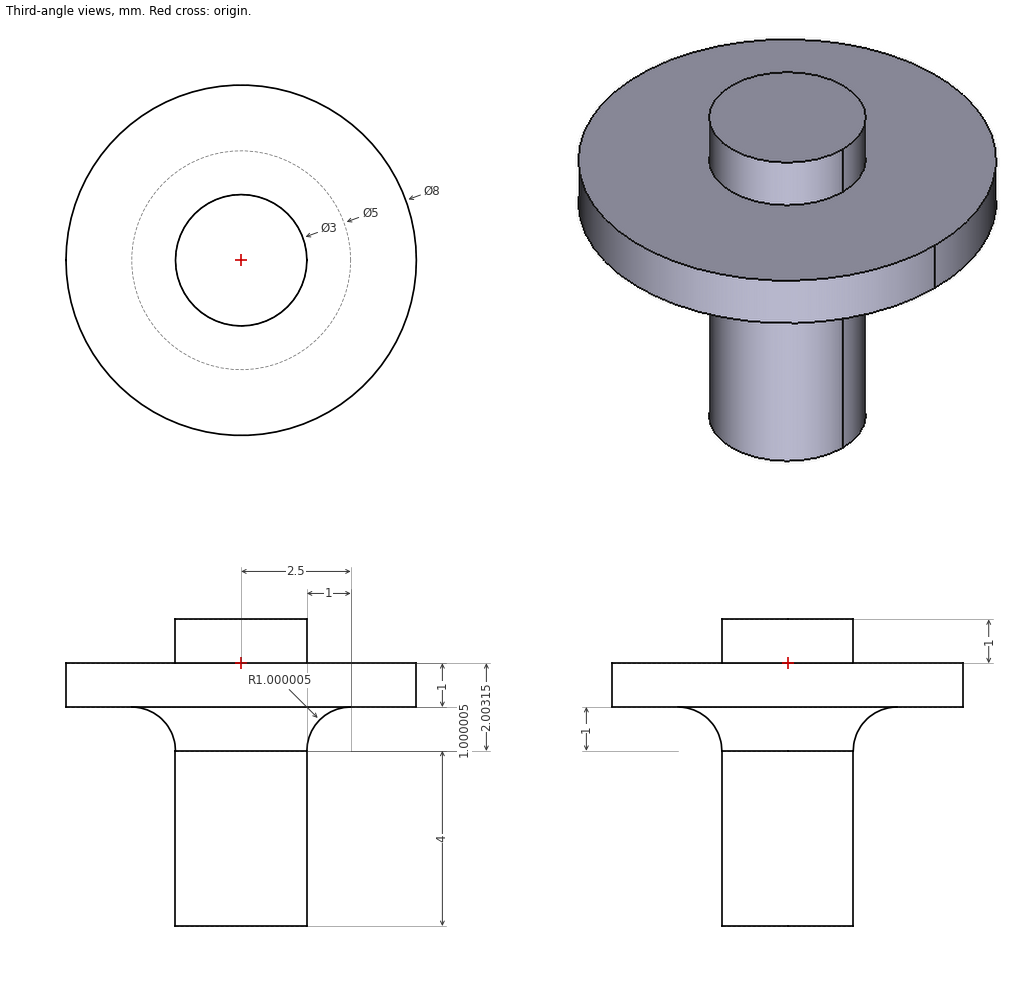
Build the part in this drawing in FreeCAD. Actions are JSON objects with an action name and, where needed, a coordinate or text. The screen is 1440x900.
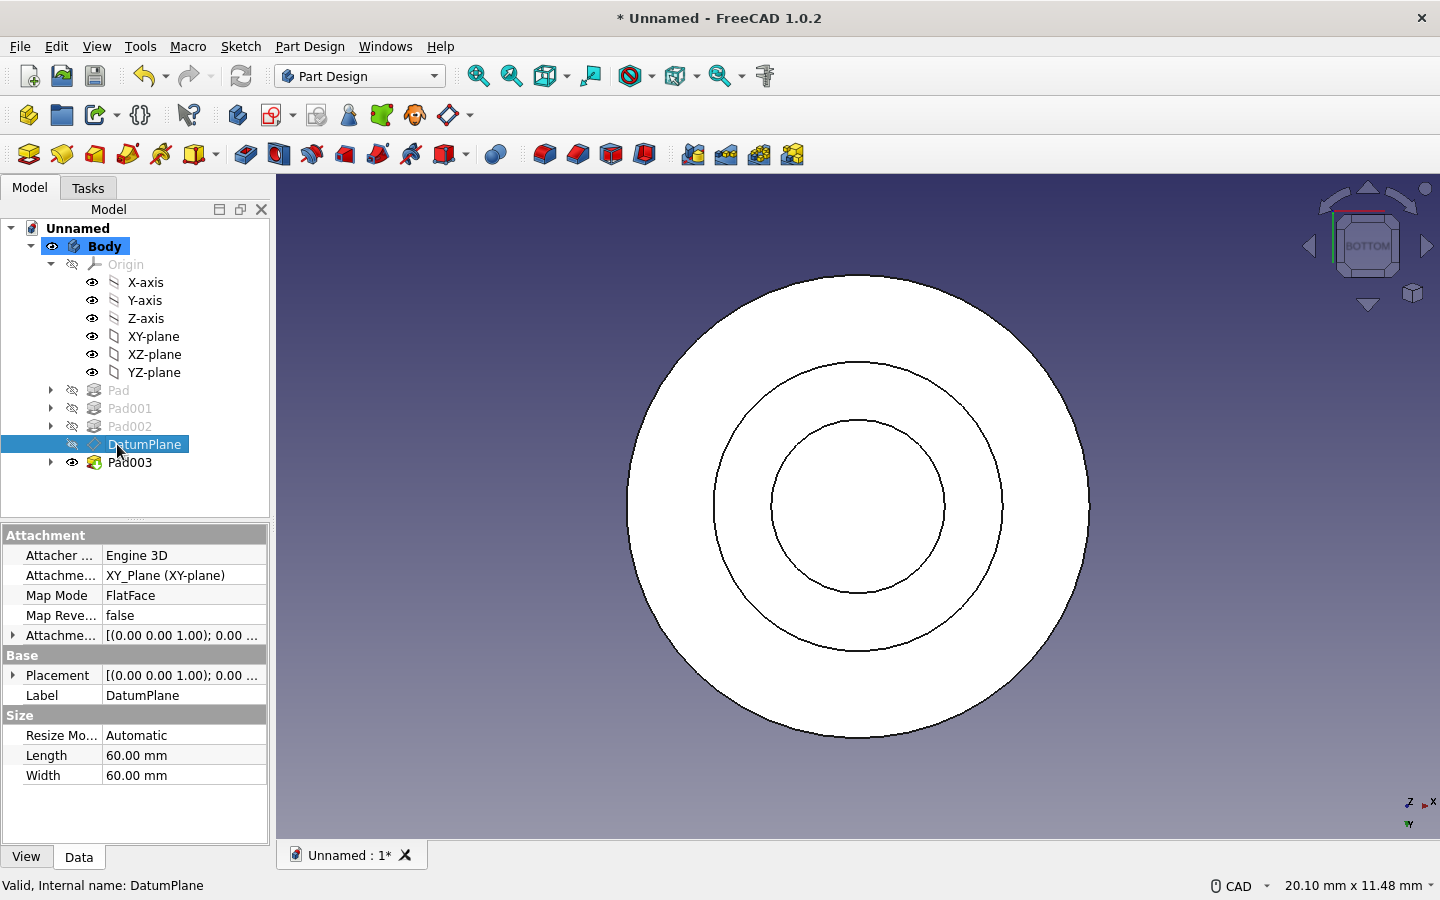
{"action": "left_click", "coordinate": [316, 799]}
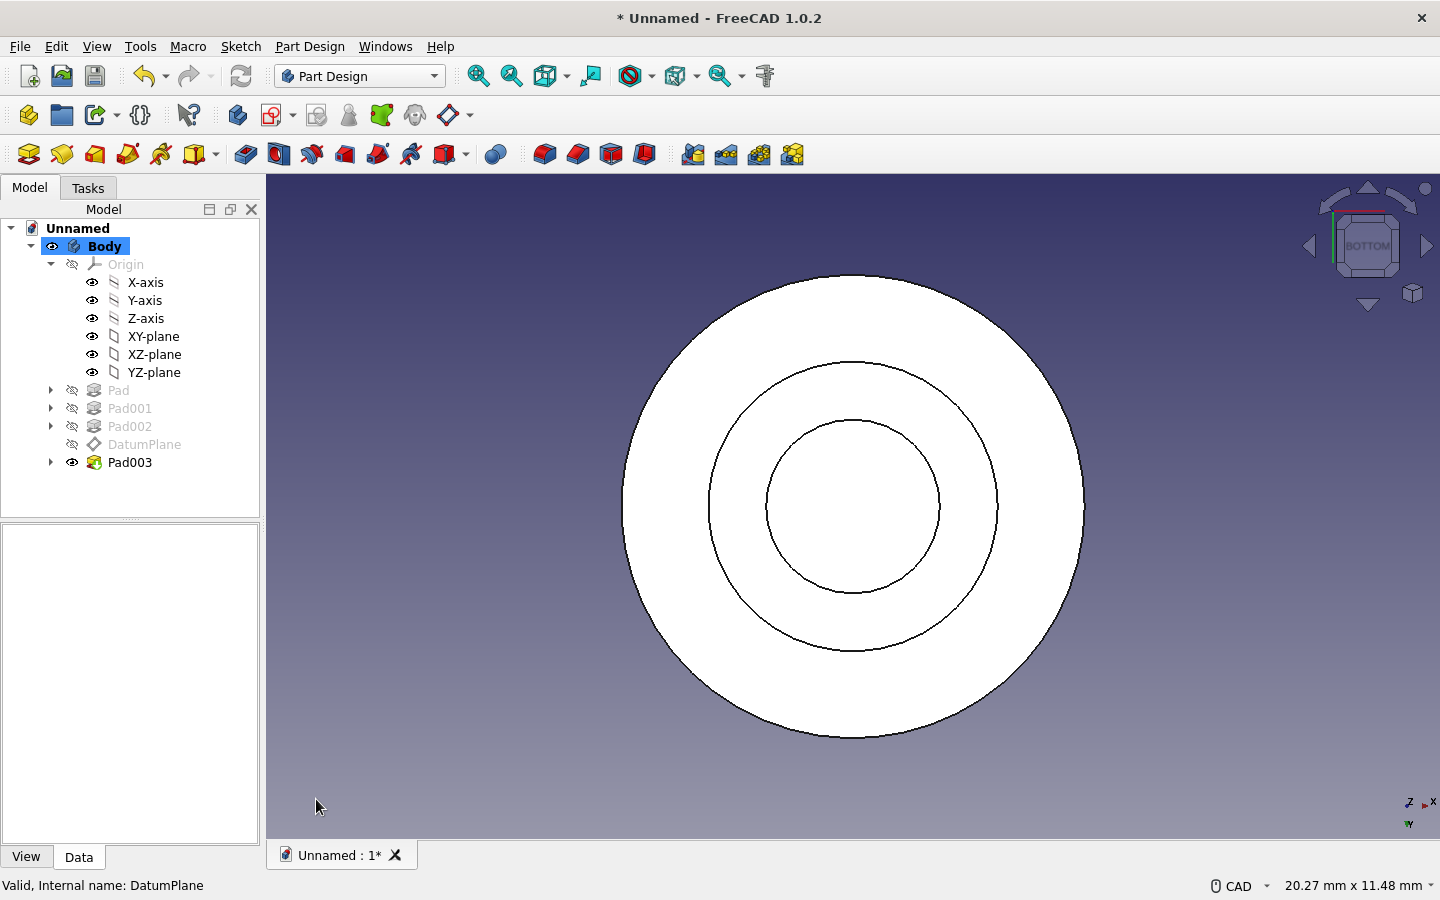
{"action": "left_click", "coordinate": [270, 116]}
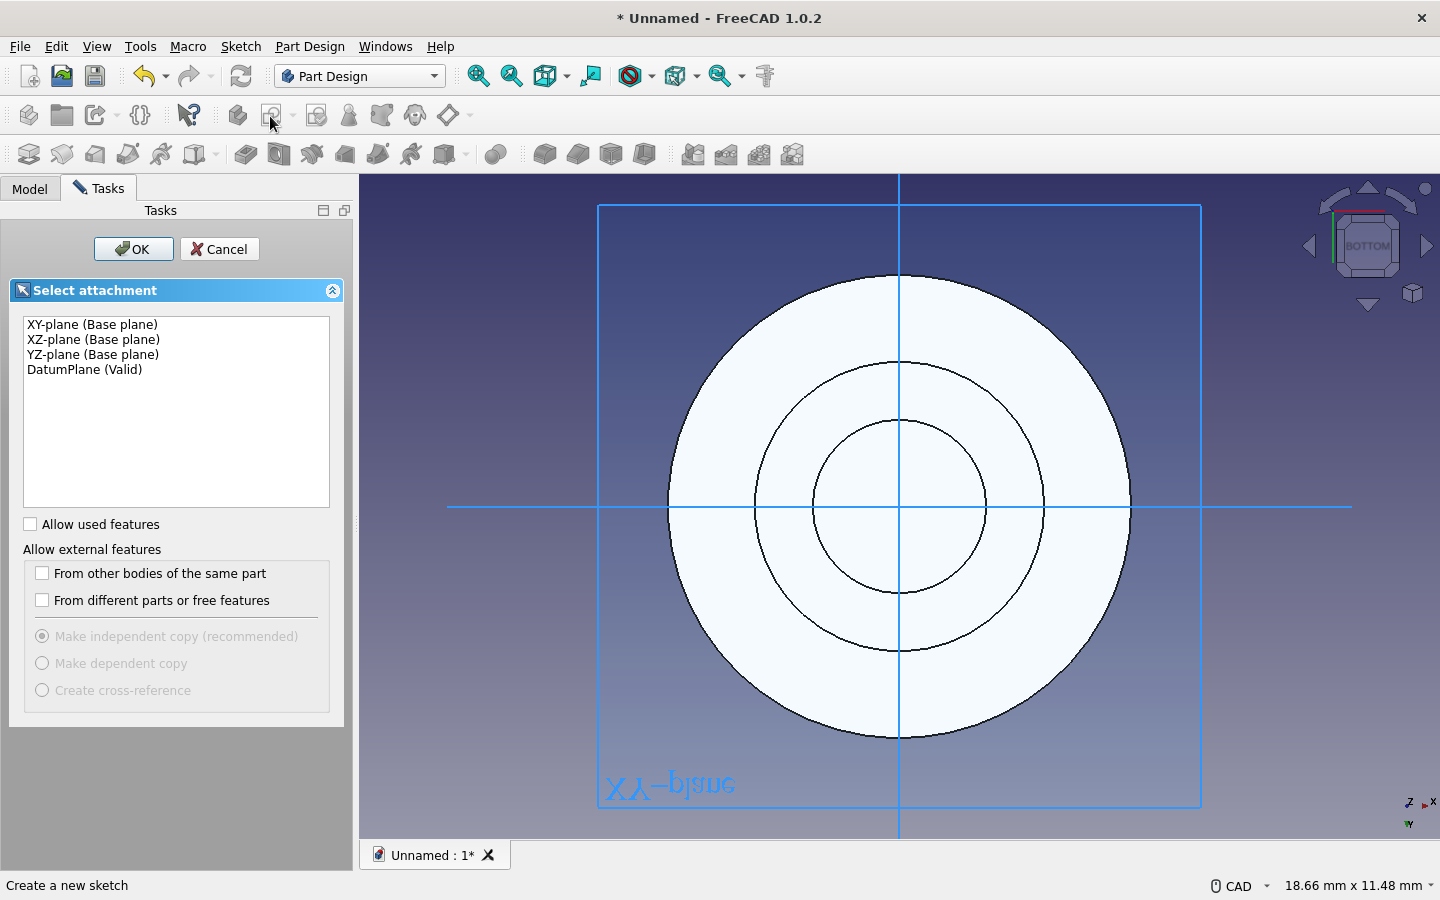
{"action": "left_click", "coordinate": [84, 340]}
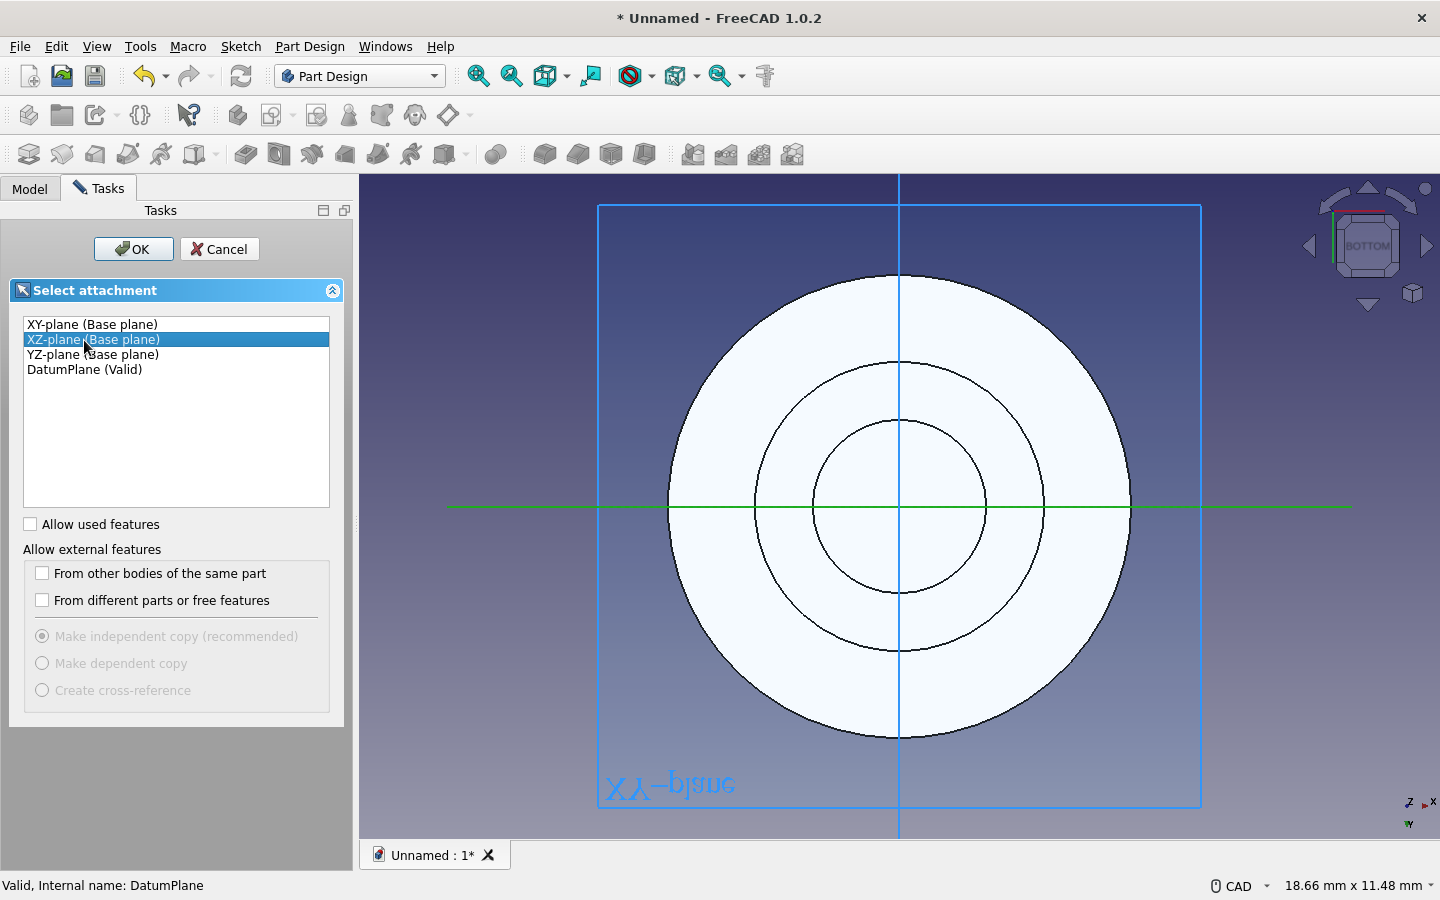
{"action": "left_click", "coordinate": [134, 249]}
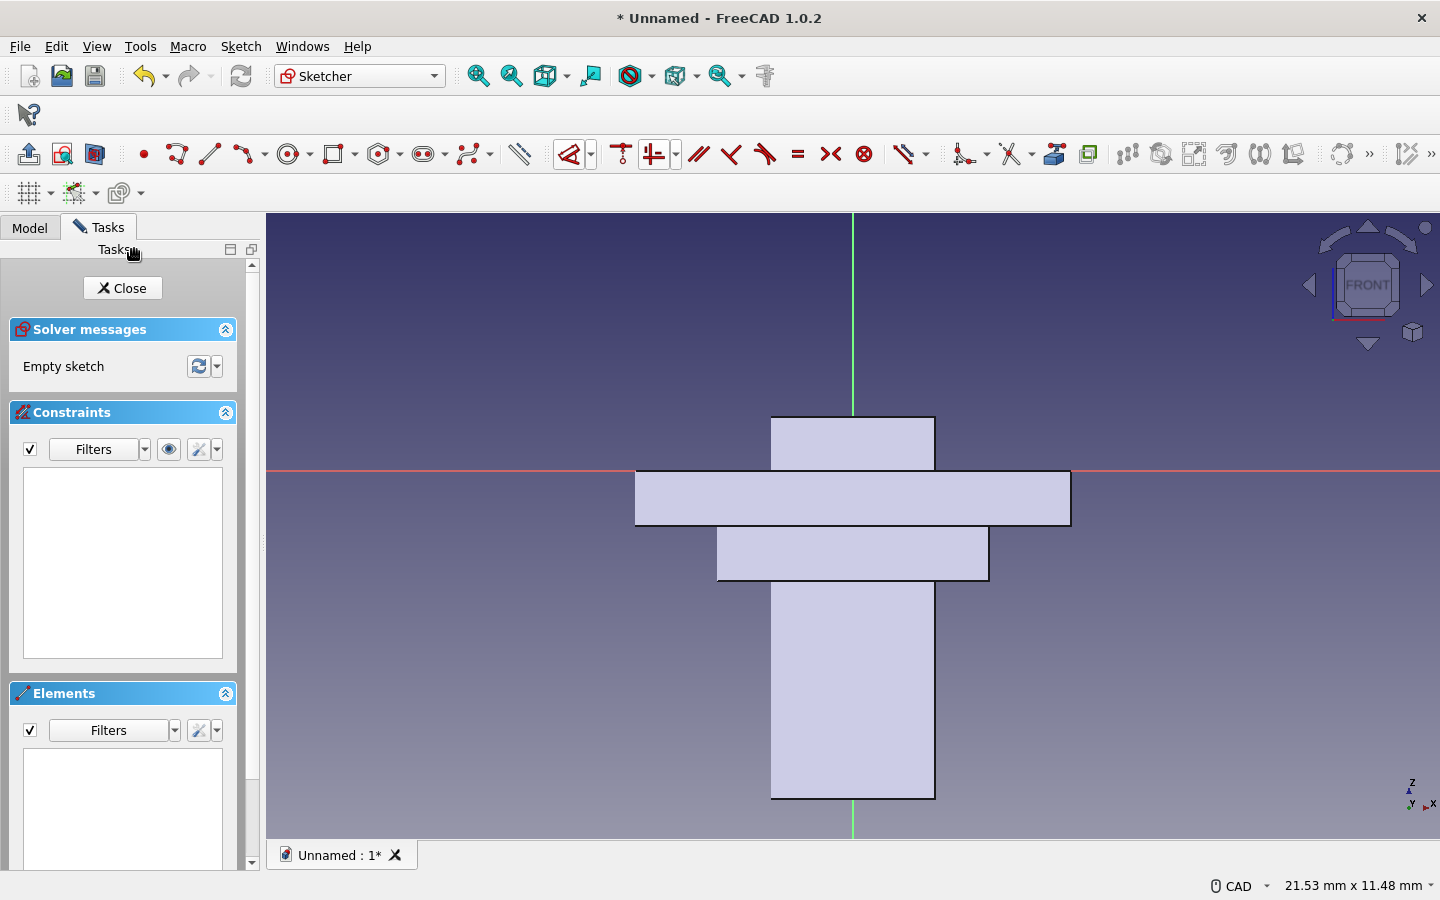
{"action": "key", "text": "q s"}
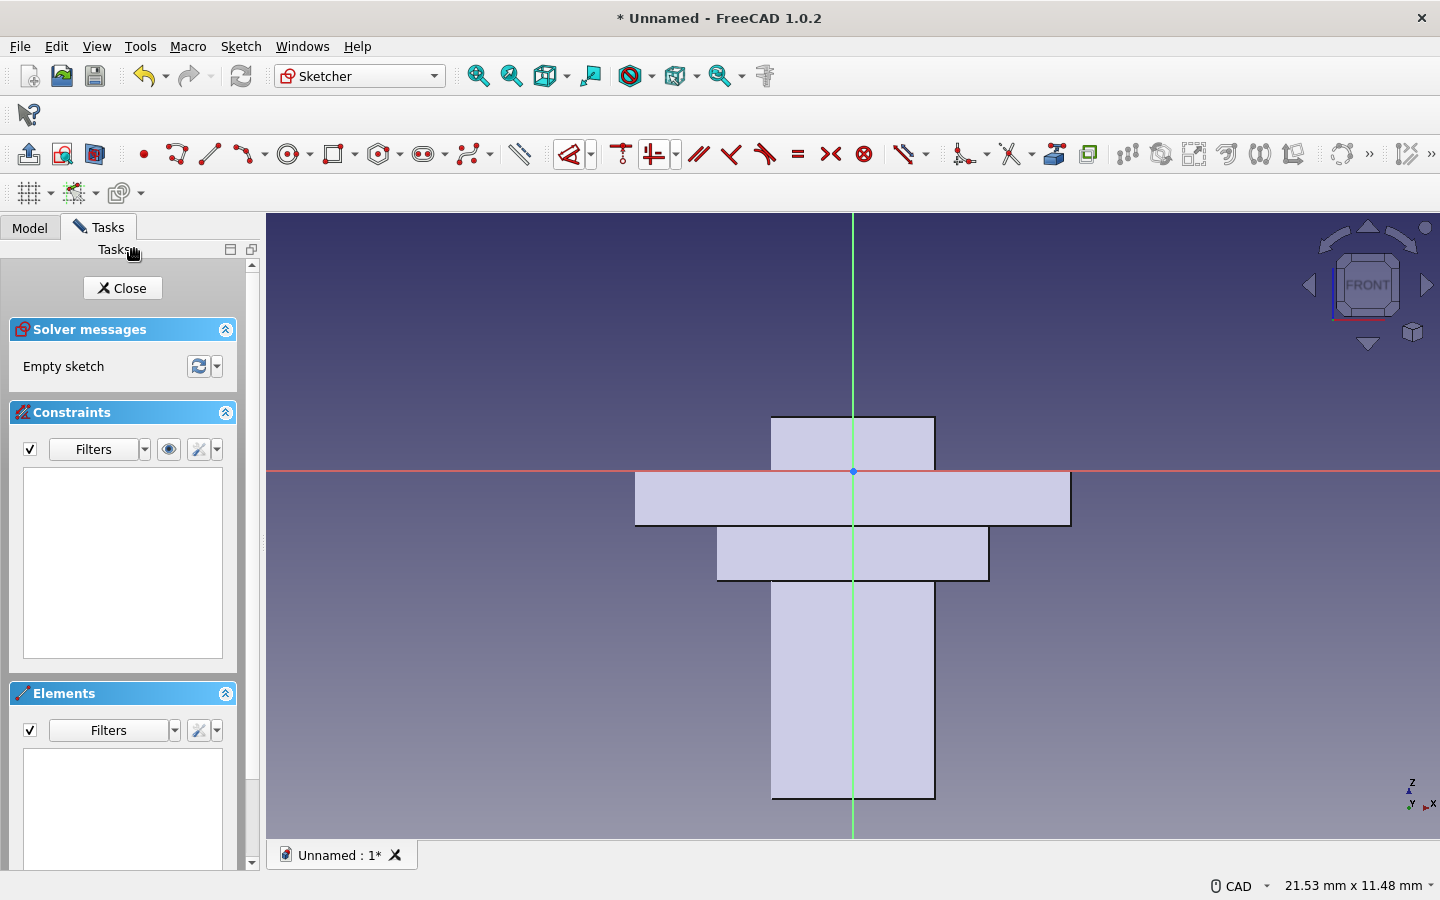
{"action": "scroll", "coordinate": [966, 526], "scroll_direction": "up", "scroll_amount": 7}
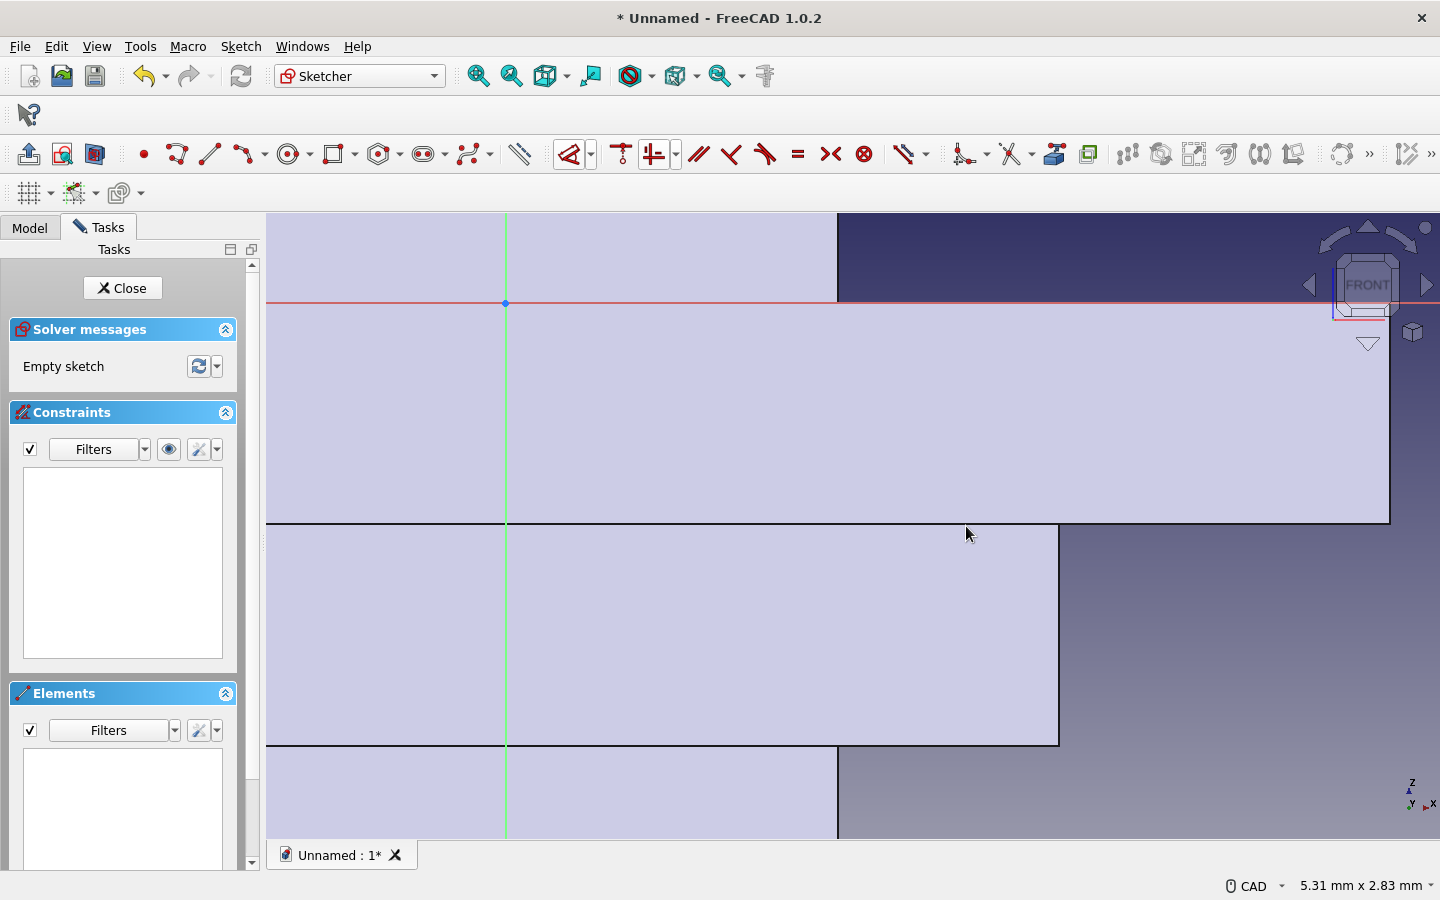
{"action": "left_click", "coordinate": [177, 154]}